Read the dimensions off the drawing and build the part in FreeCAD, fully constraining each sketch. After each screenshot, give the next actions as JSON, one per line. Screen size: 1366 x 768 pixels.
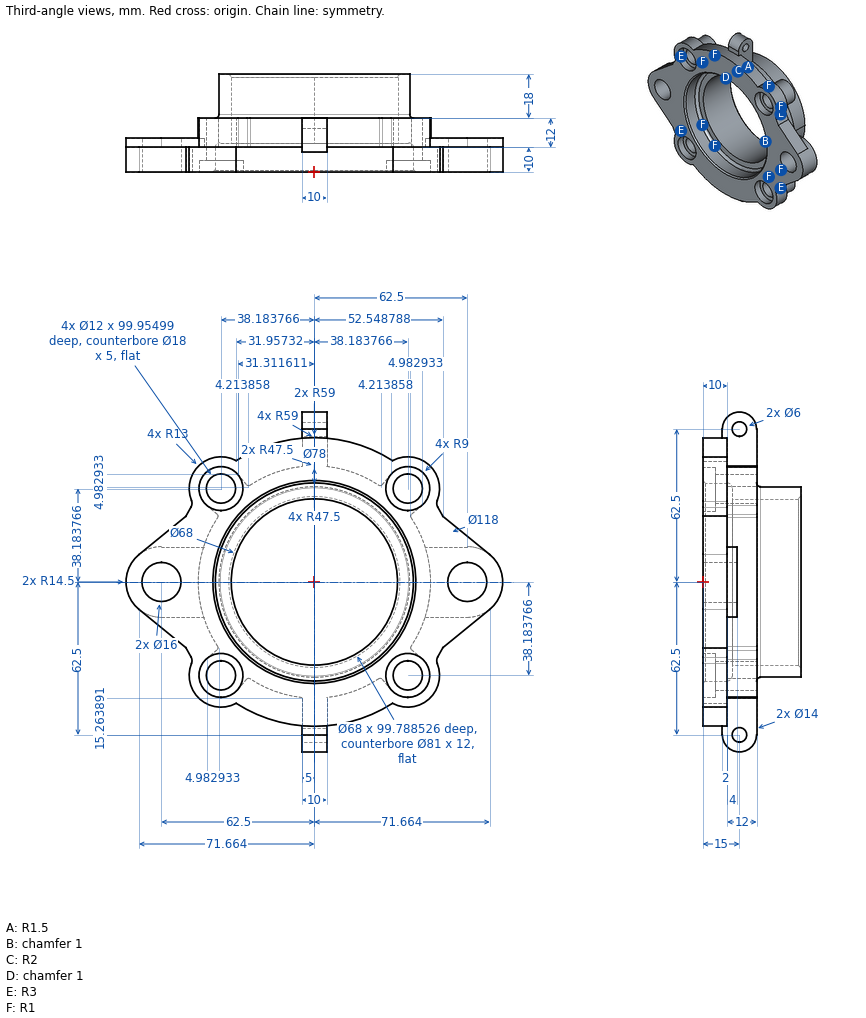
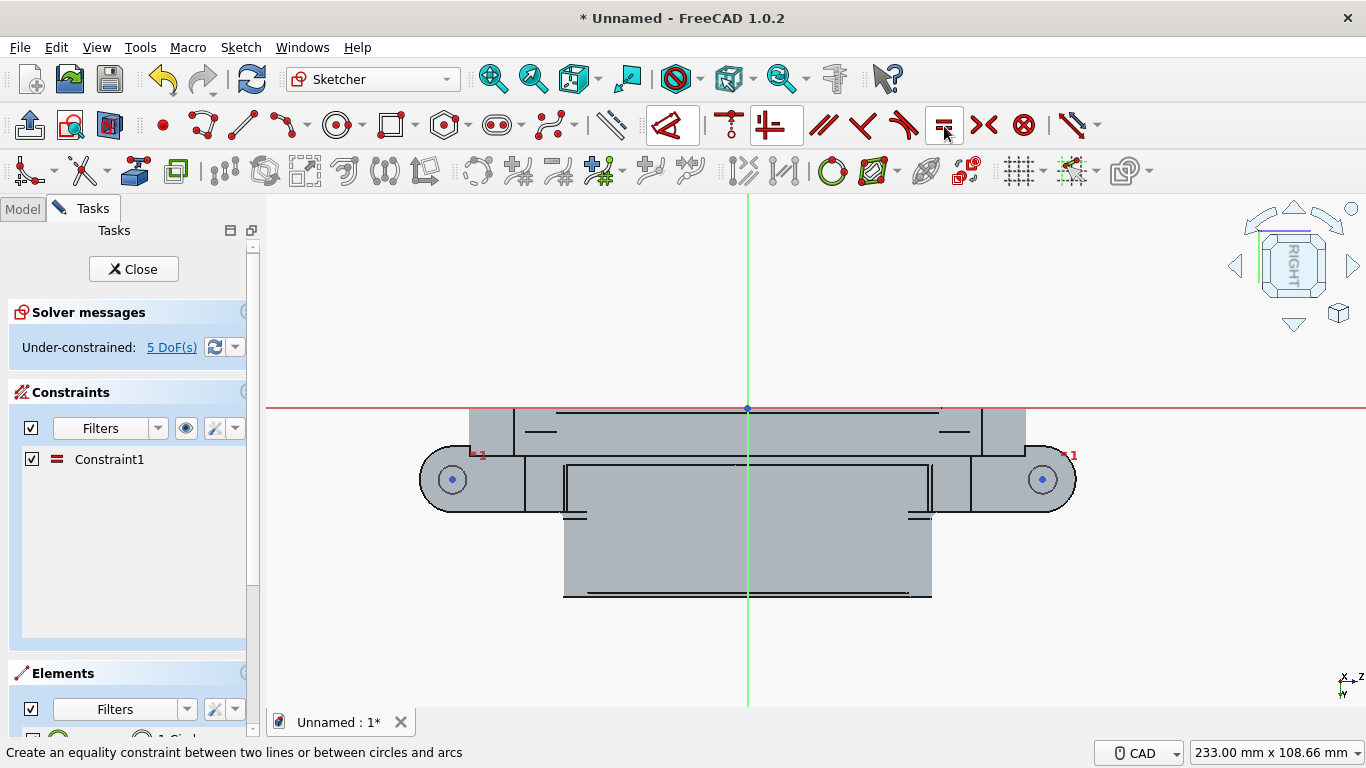
{"action": "left_click", "coordinate": [1043, 480]}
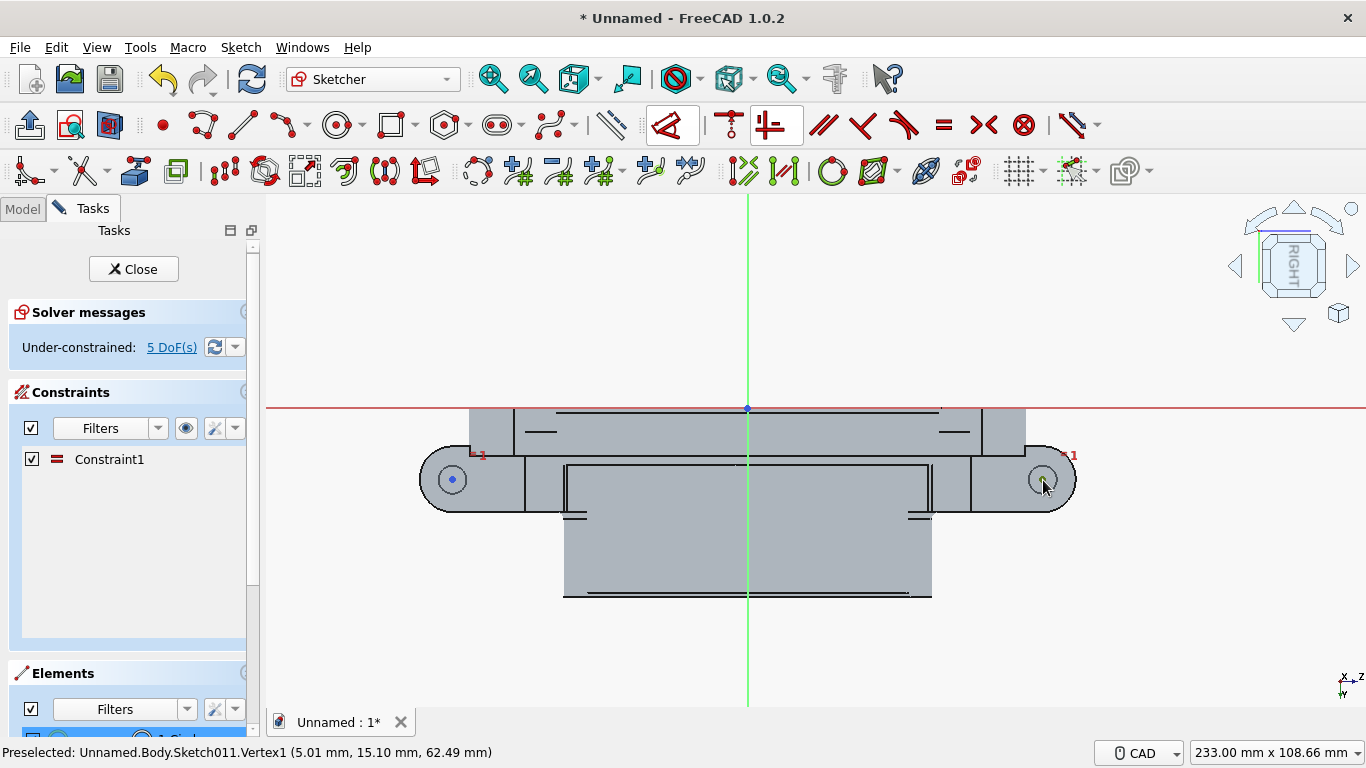
{"action": "left_click", "coordinate": [453, 480]}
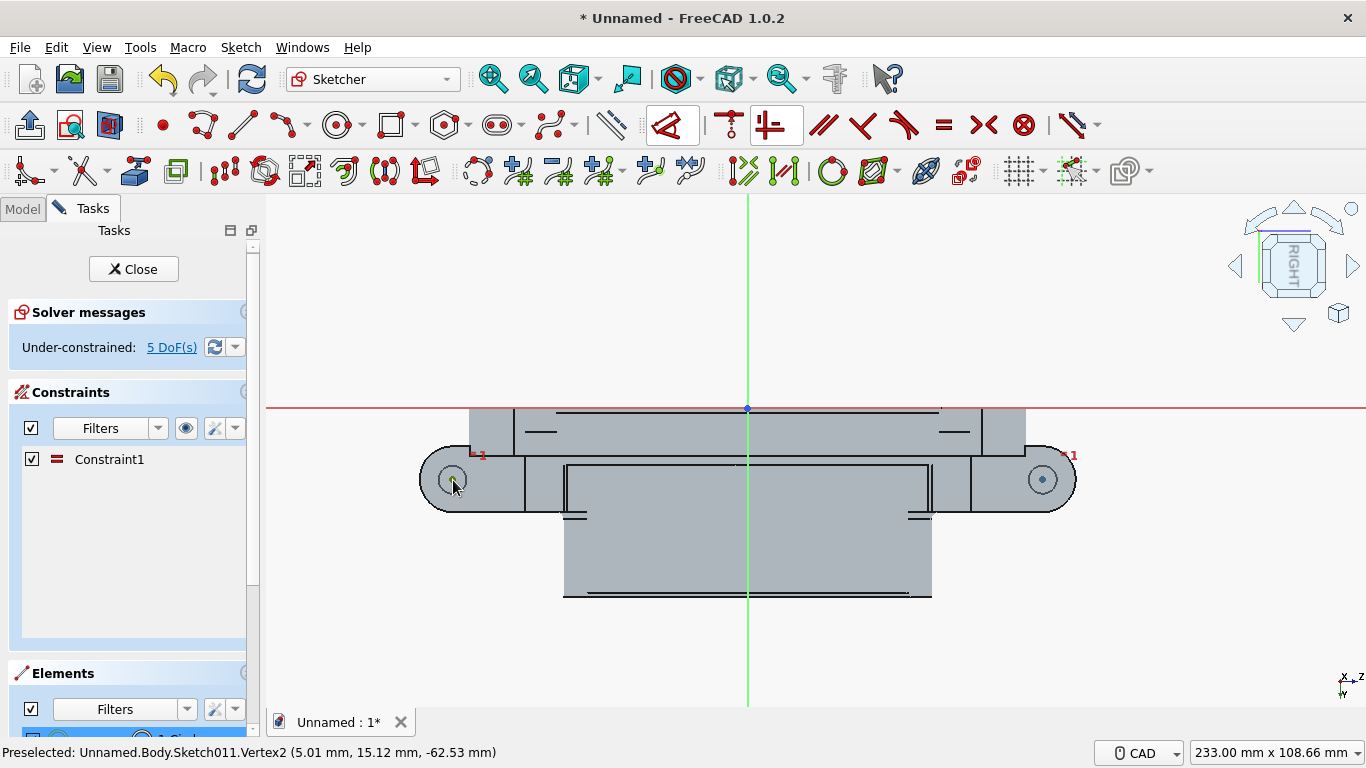
{"action": "left_click", "coordinate": [798, 126]}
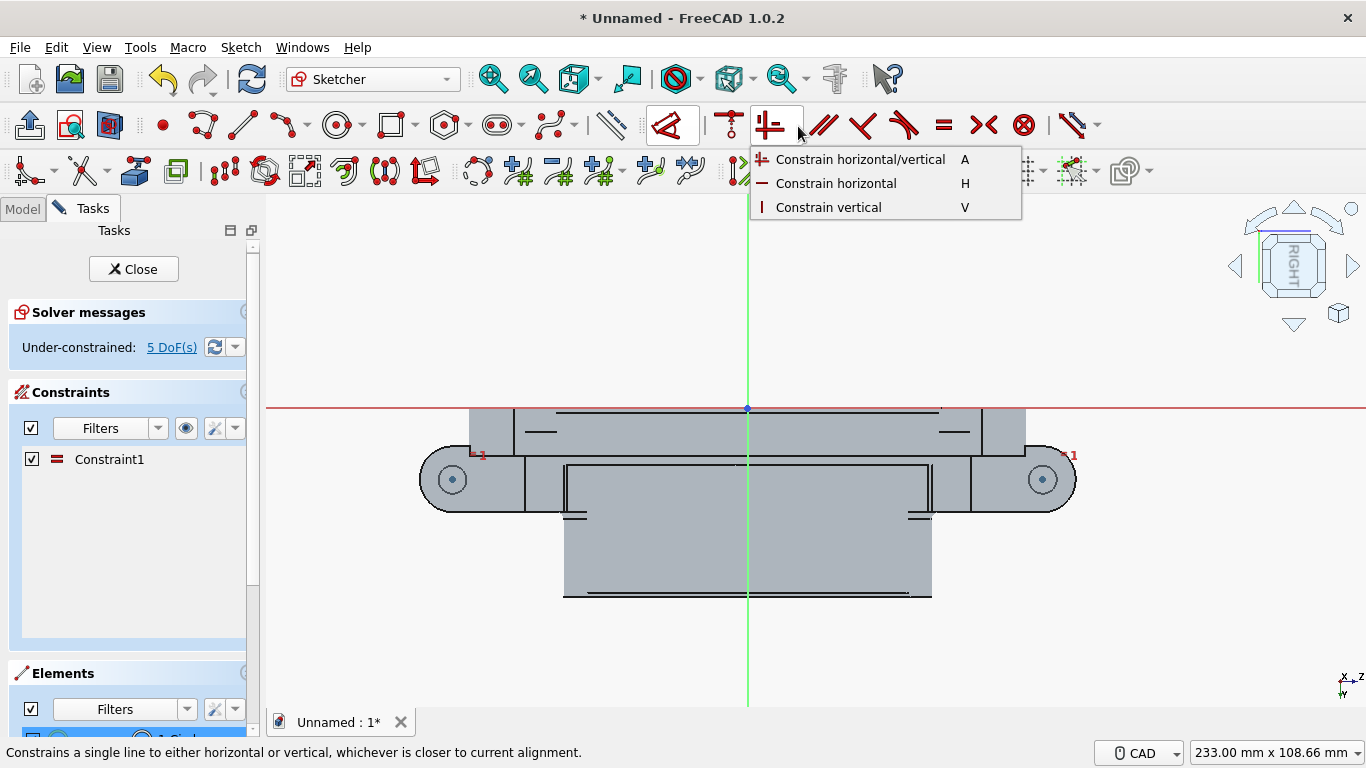
{"action": "left_click", "coordinate": [886, 183]}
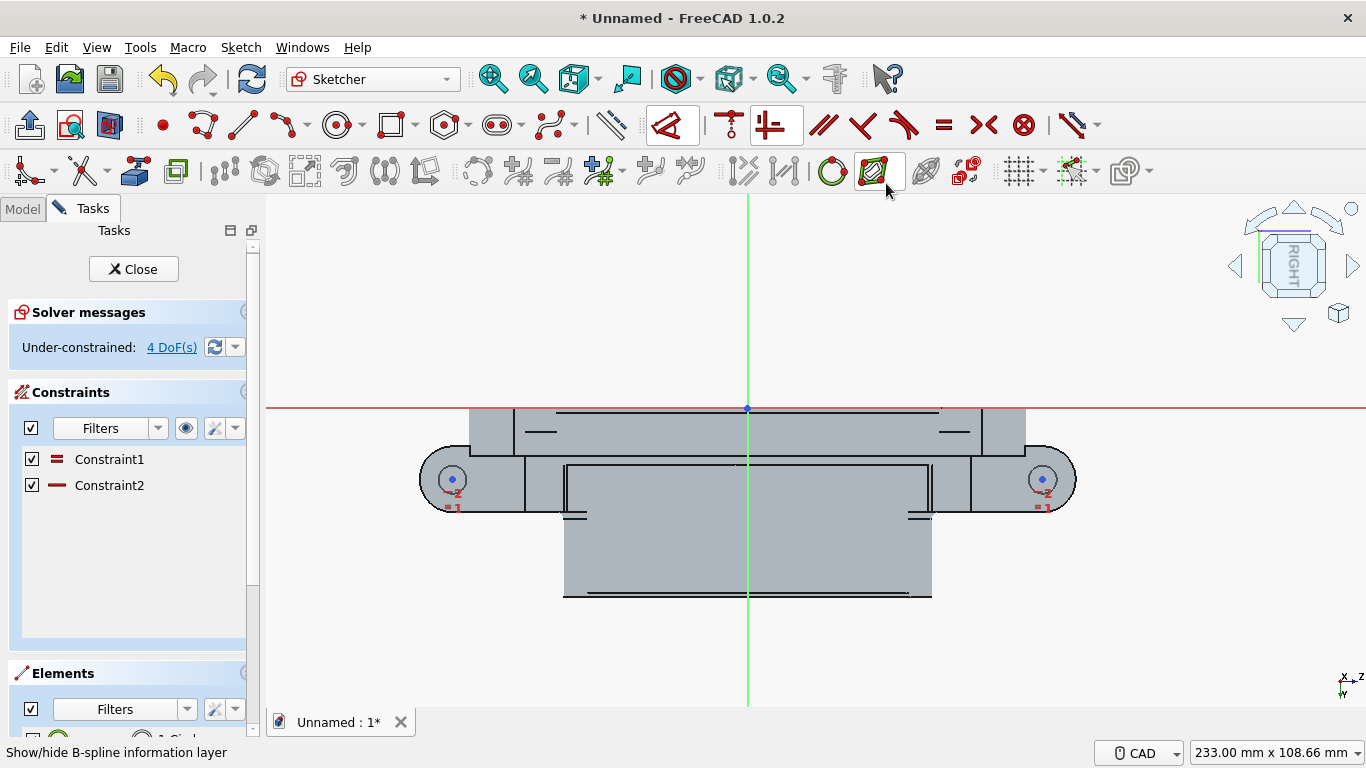
{"action": "scroll", "coordinate": [1053, 470], "scroll_direction": "up", "scroll_amount": 2}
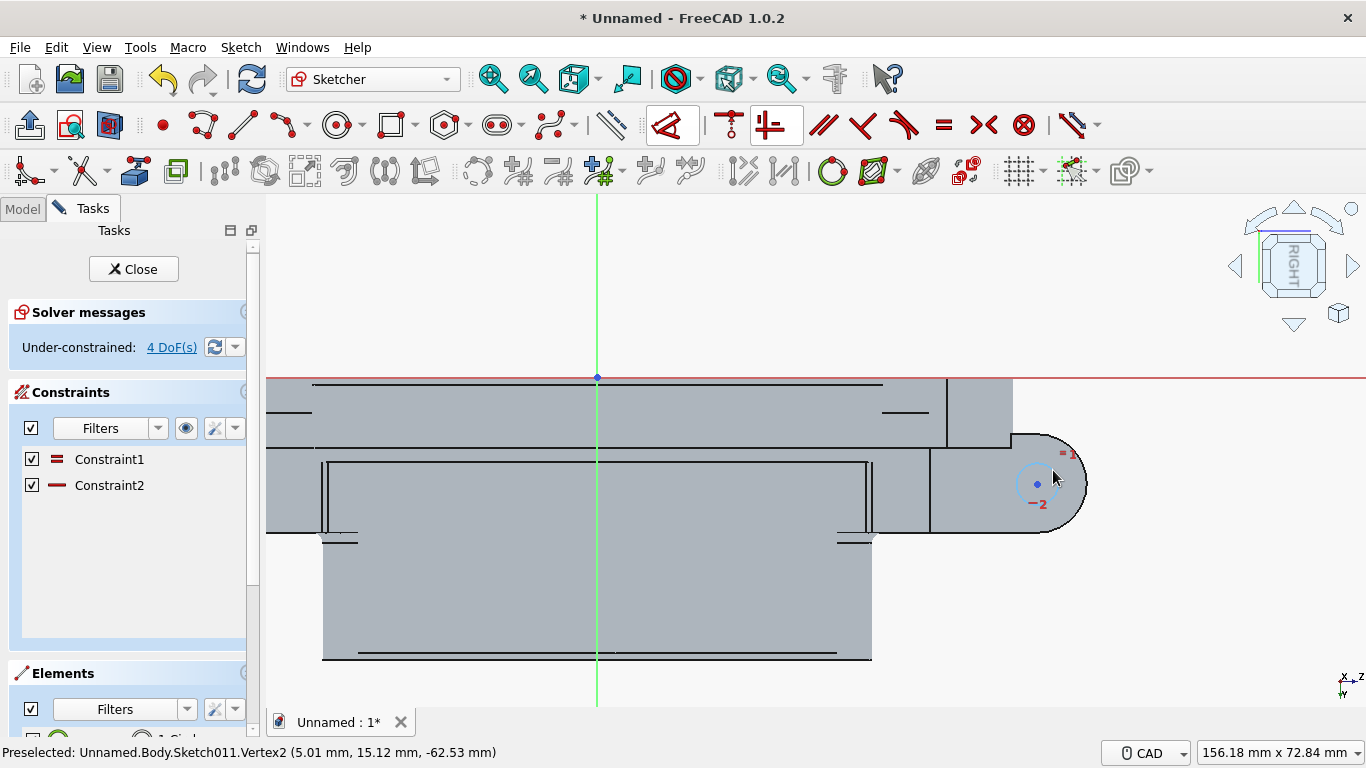
{"action": "left_click", "coordinate": [1052, 469]}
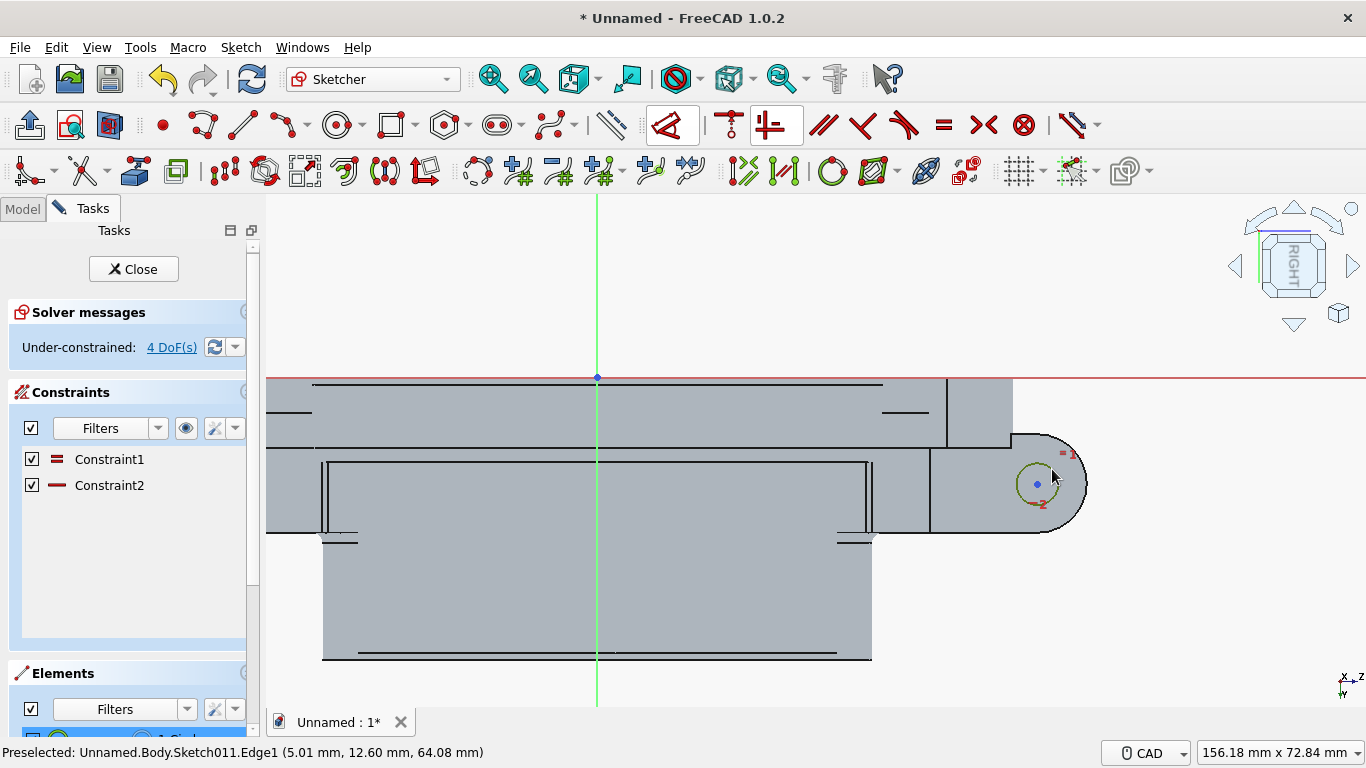
{"action": "key", "text": "k o"}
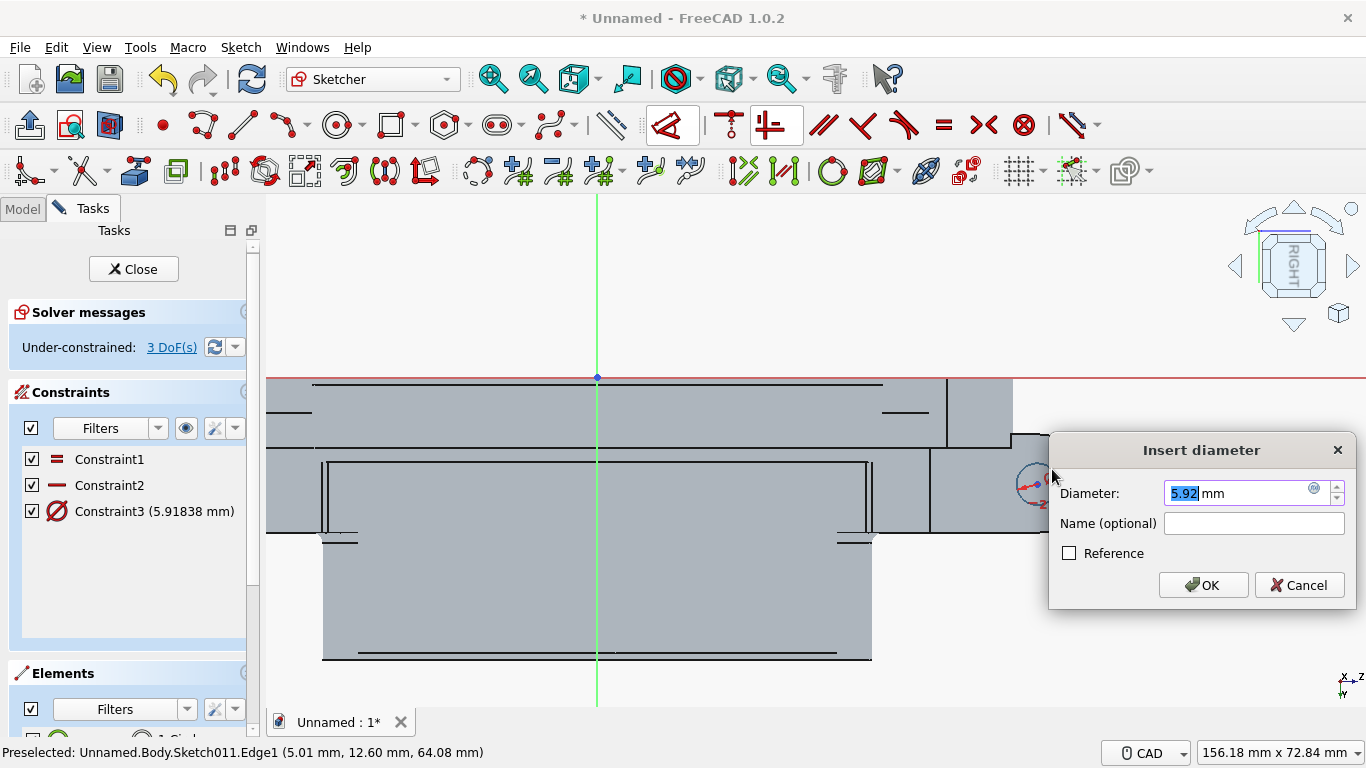
{"action": "type", "text": "6"}
{"action": "key", "text": "Return"}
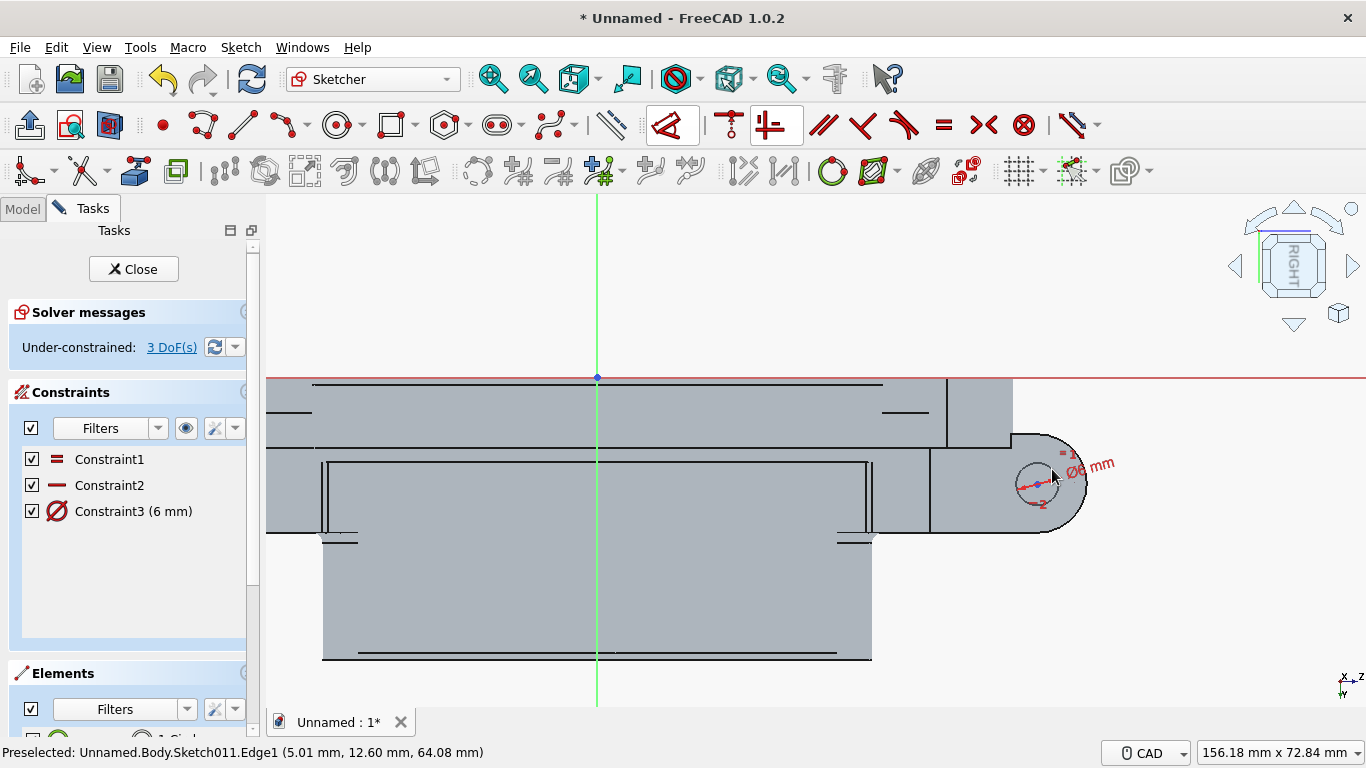
{"action": "left_click", "coordinate": [1037, 484]}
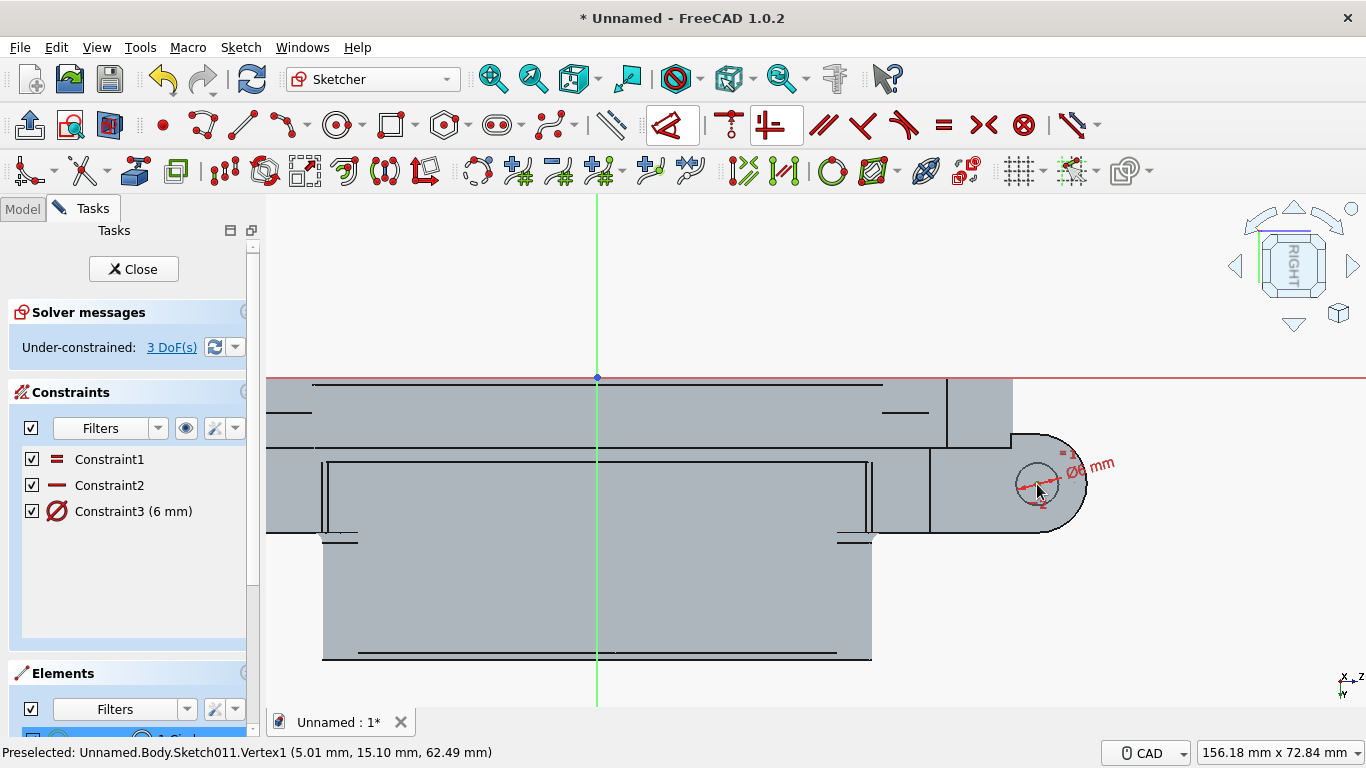
{"action": "left_click", "coordinate": [694, 126]}